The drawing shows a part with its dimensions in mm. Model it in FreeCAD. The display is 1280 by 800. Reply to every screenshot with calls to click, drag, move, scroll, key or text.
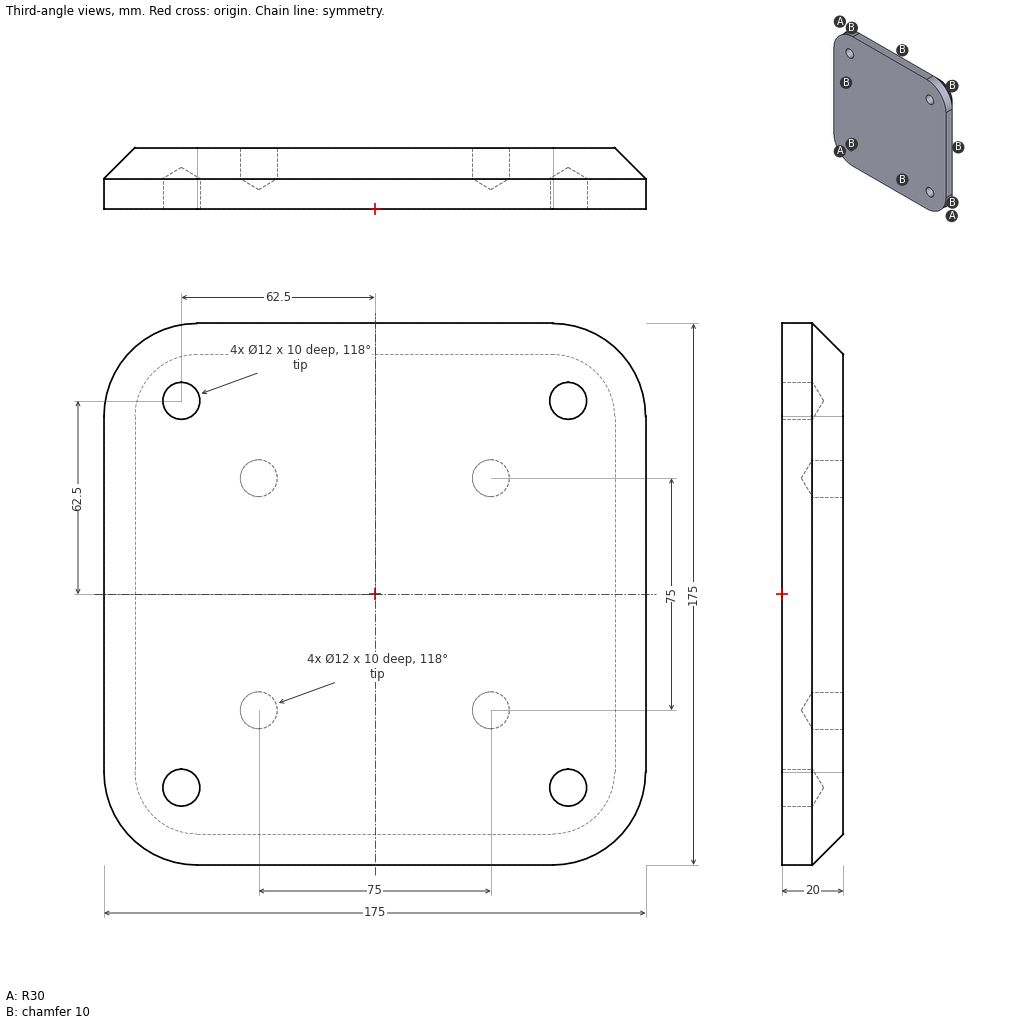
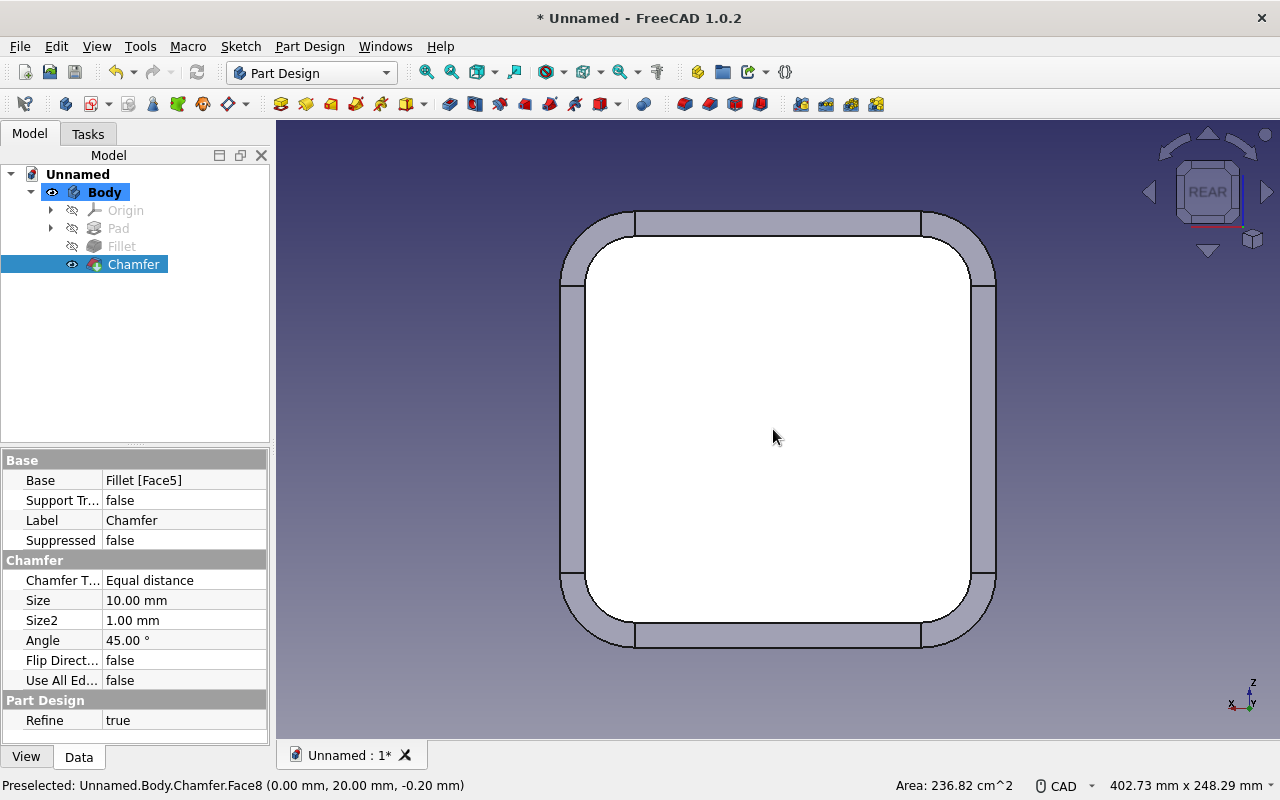
click(90, 104)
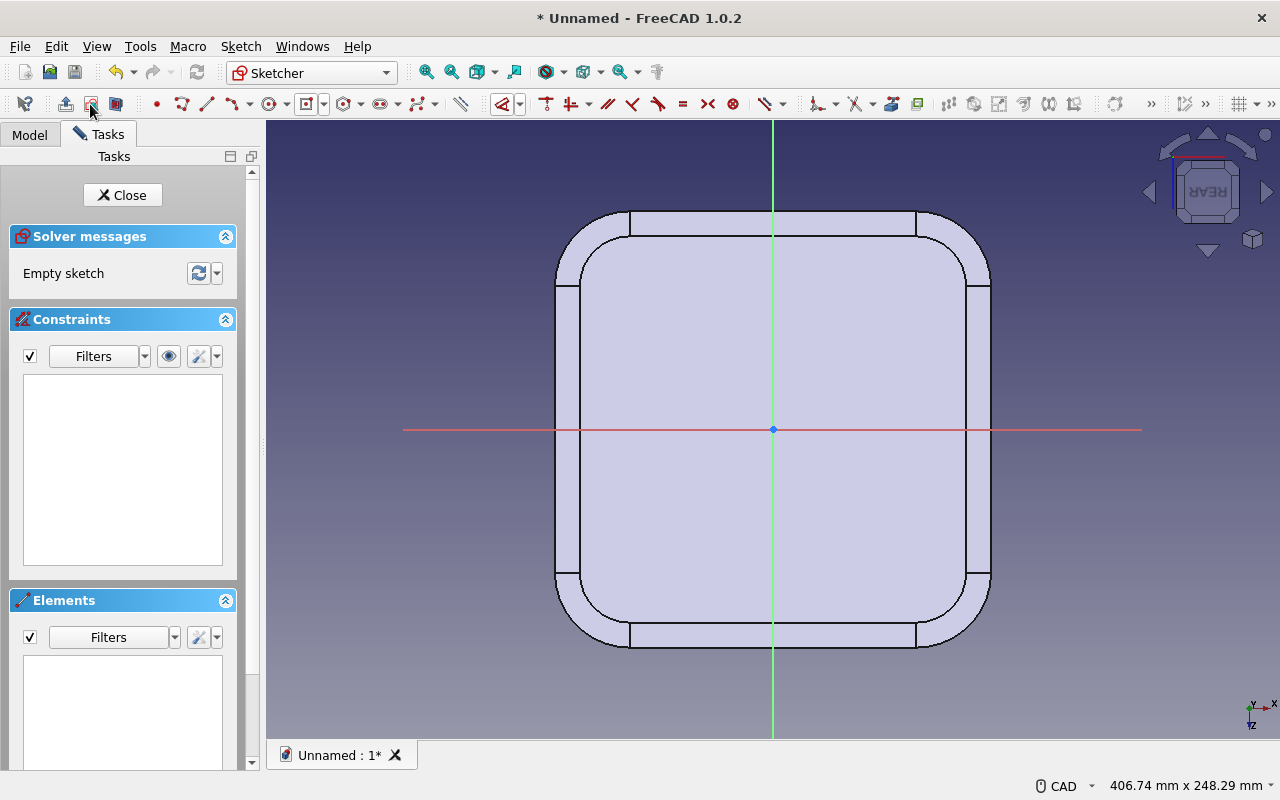
scroll(856, 429, up, 3)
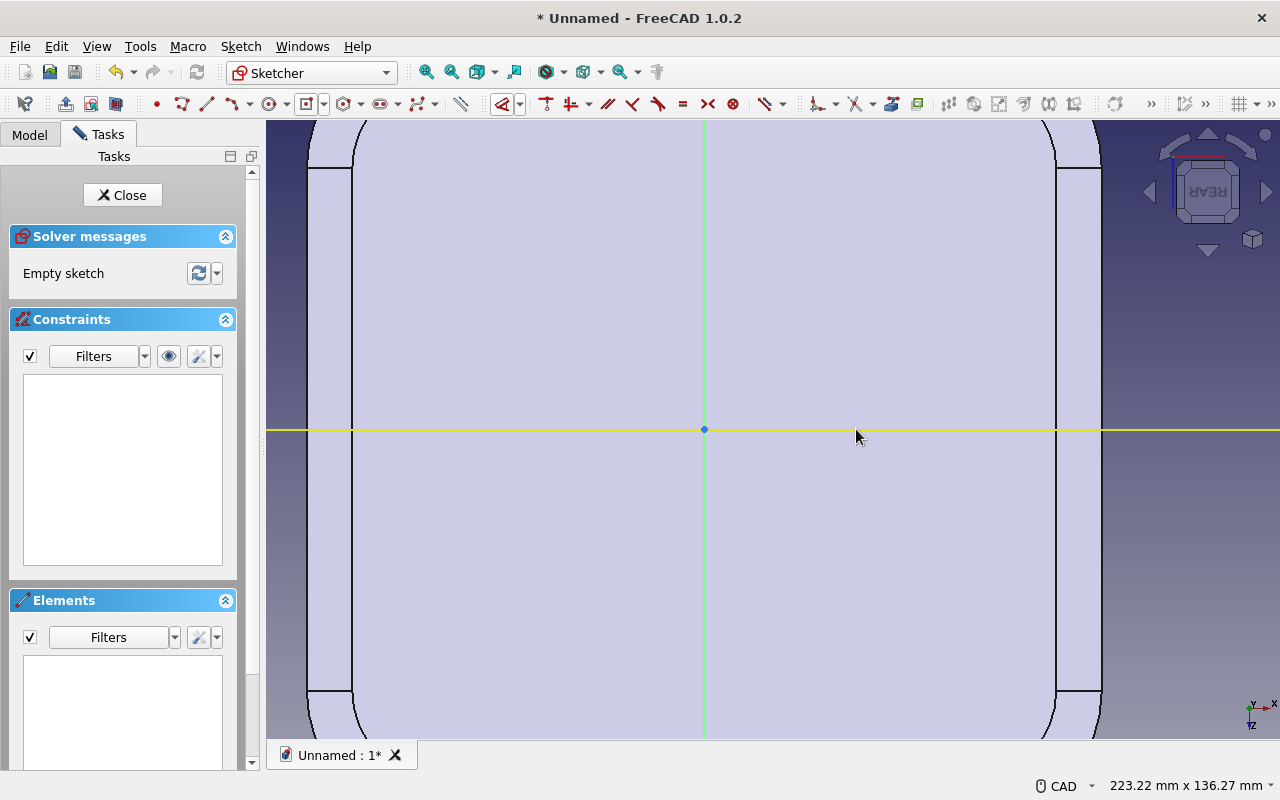
click(268, 104)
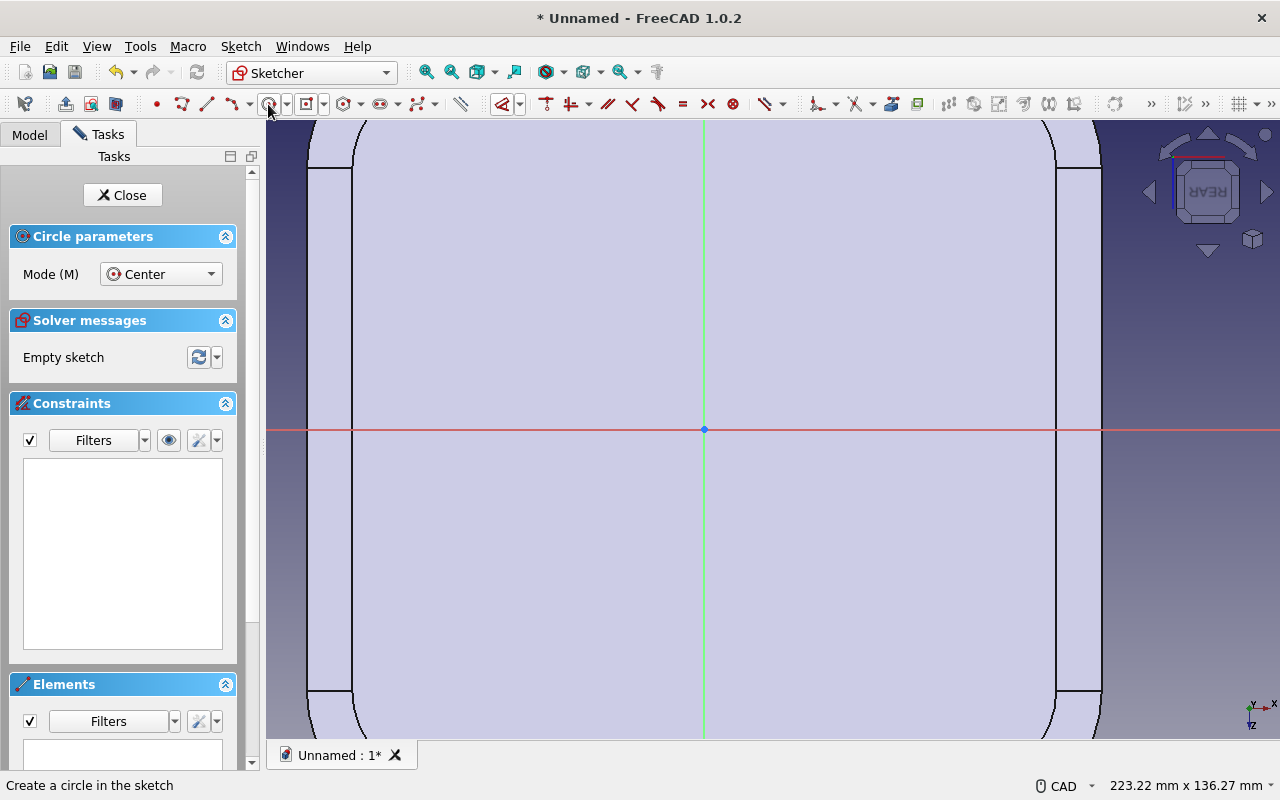
click(534, 259)
click(553, 240)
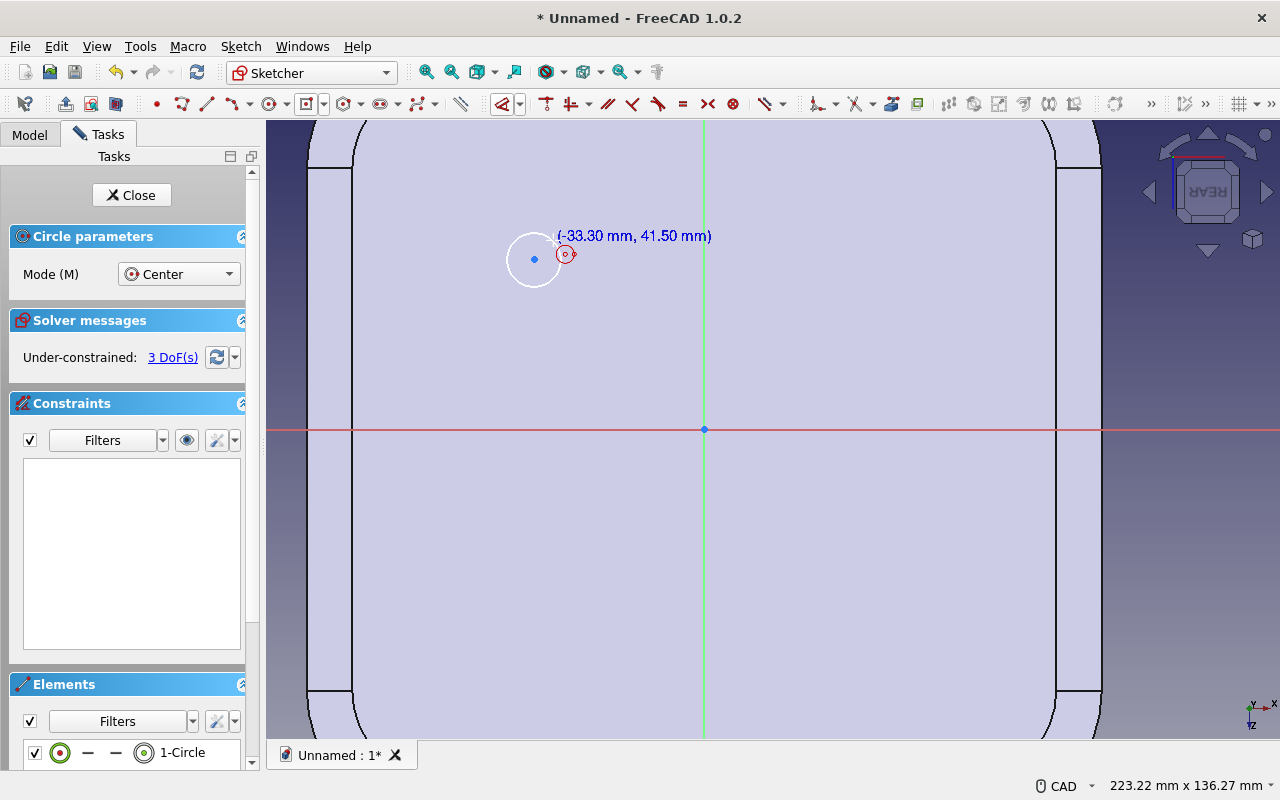
click(875, 259)
click(894, 240)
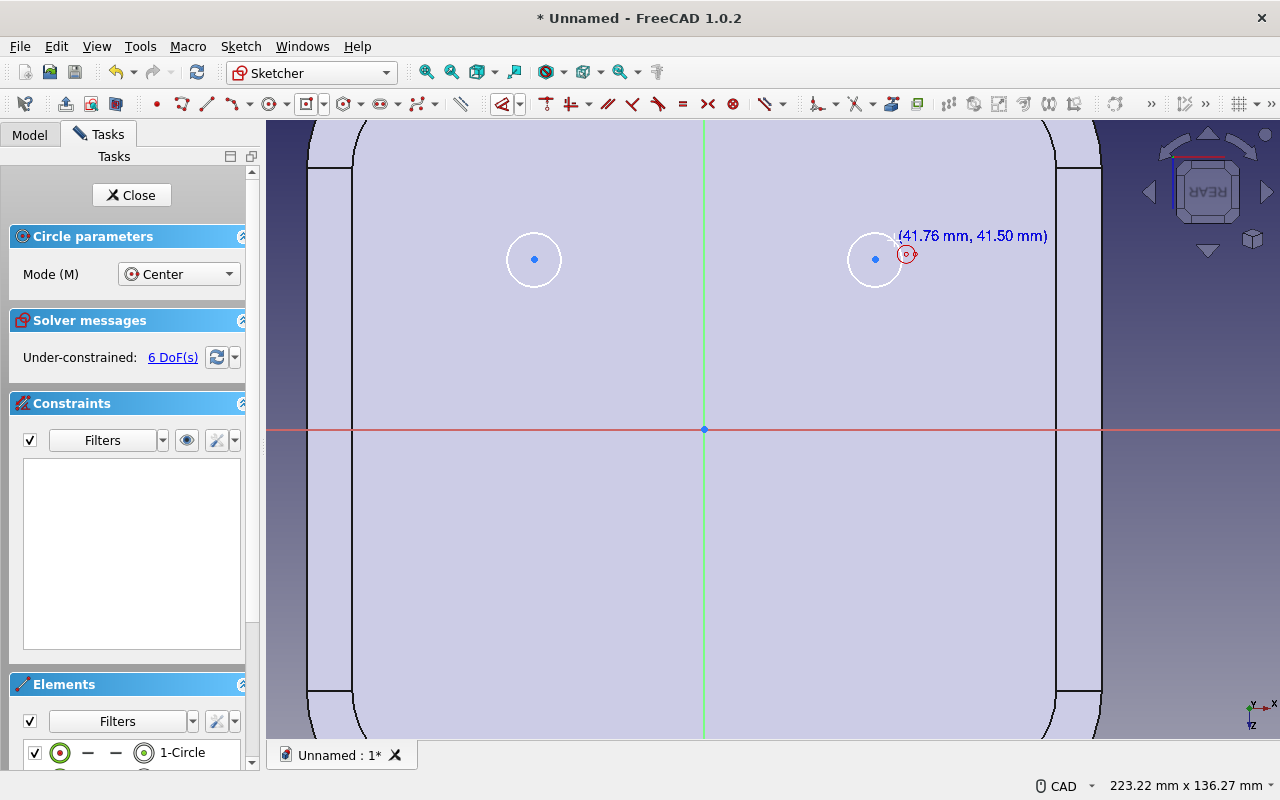
click(875, 600)
click(894, 581)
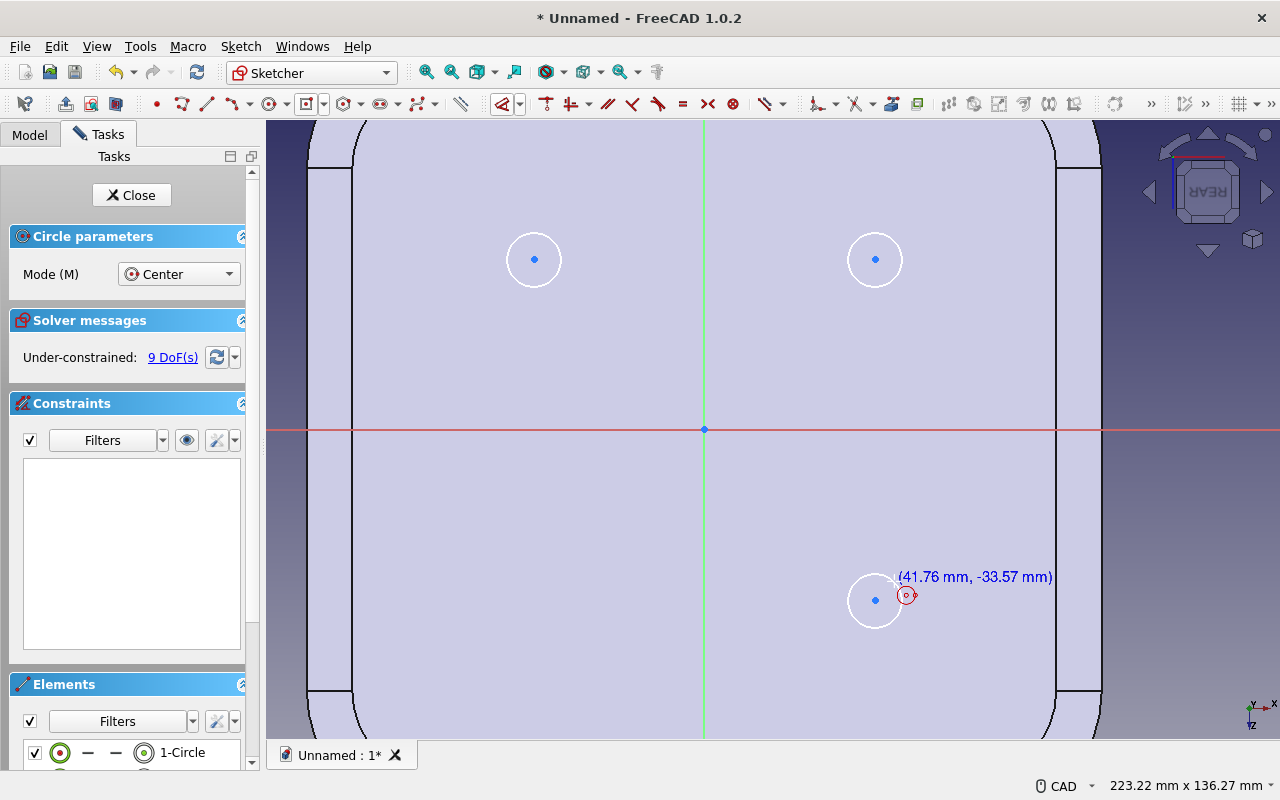
click(534, 600)
click(553, 581)
key(Escape)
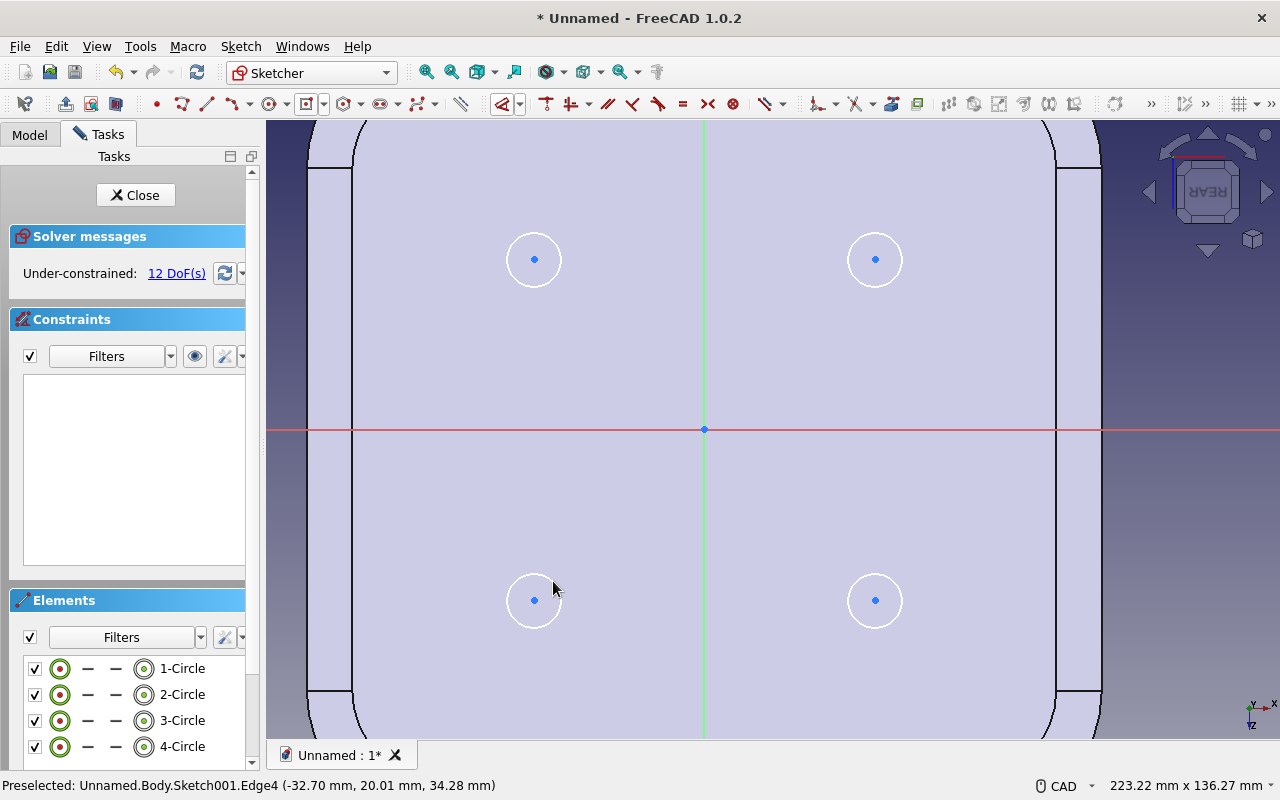
click(553, 241)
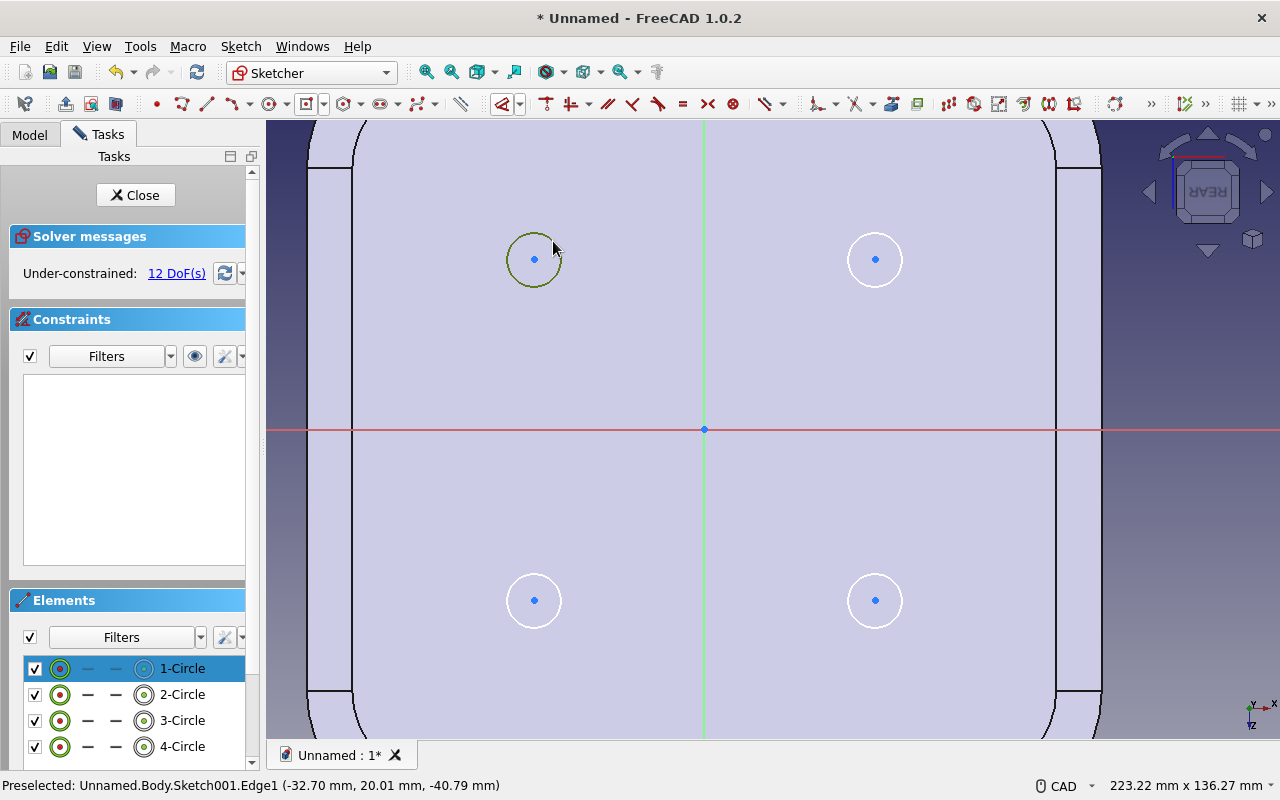
click(894, 241)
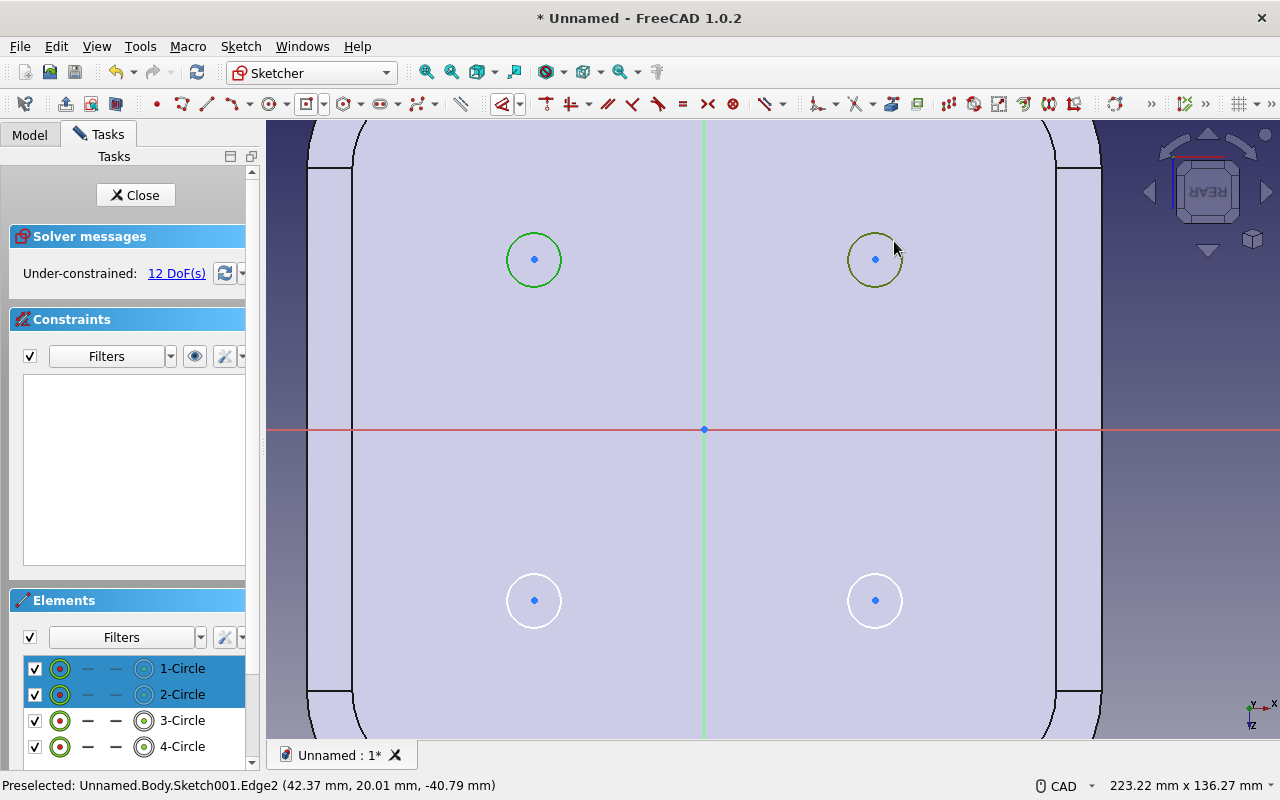
click(894, 582)